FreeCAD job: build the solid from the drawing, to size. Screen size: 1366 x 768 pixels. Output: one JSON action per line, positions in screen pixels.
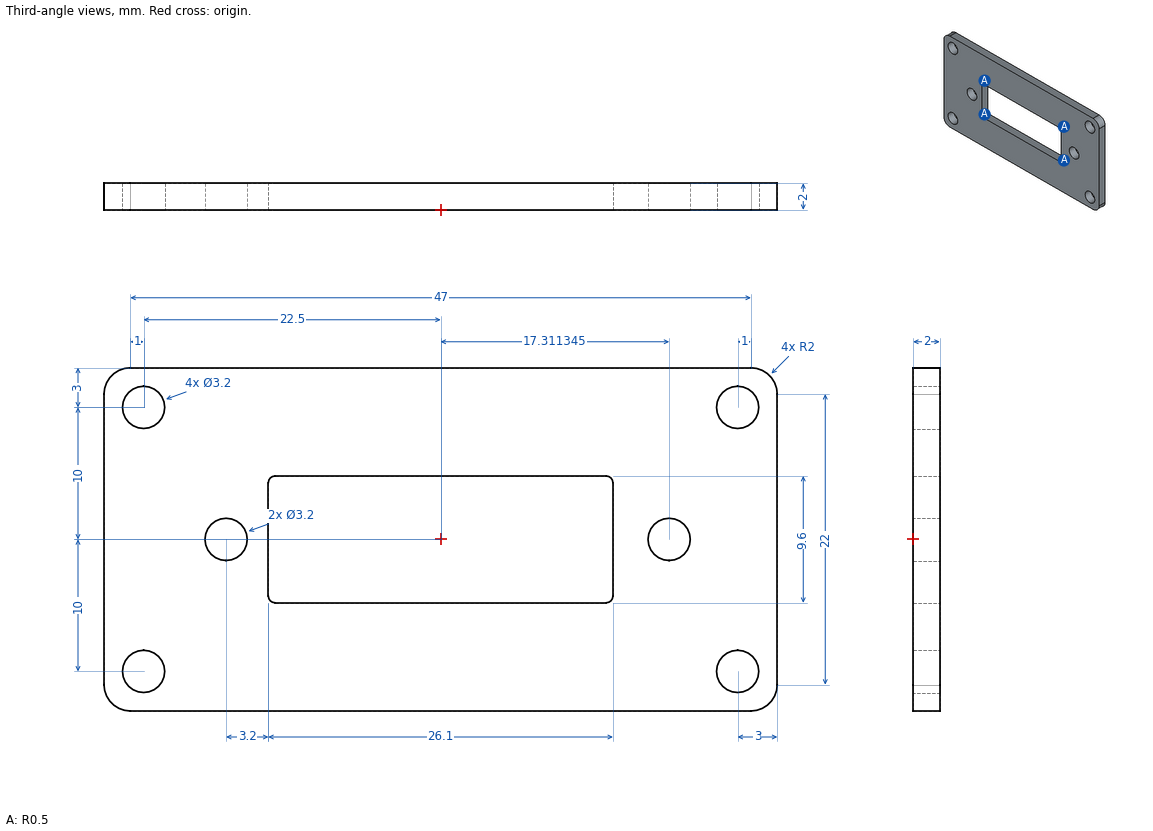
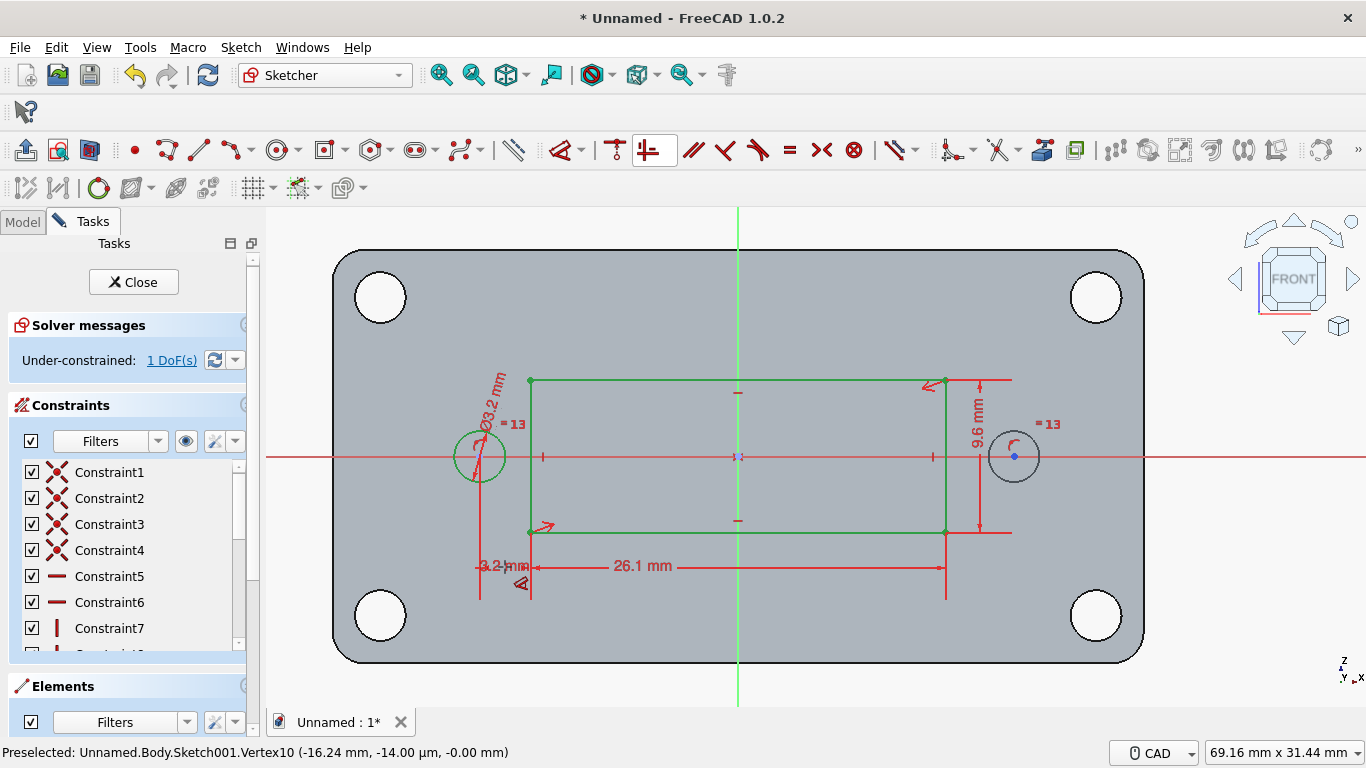
{"action": "left_click", "coordinate": [1014, 457]}
{"action": "left_click", "coordinate": [876, 491]}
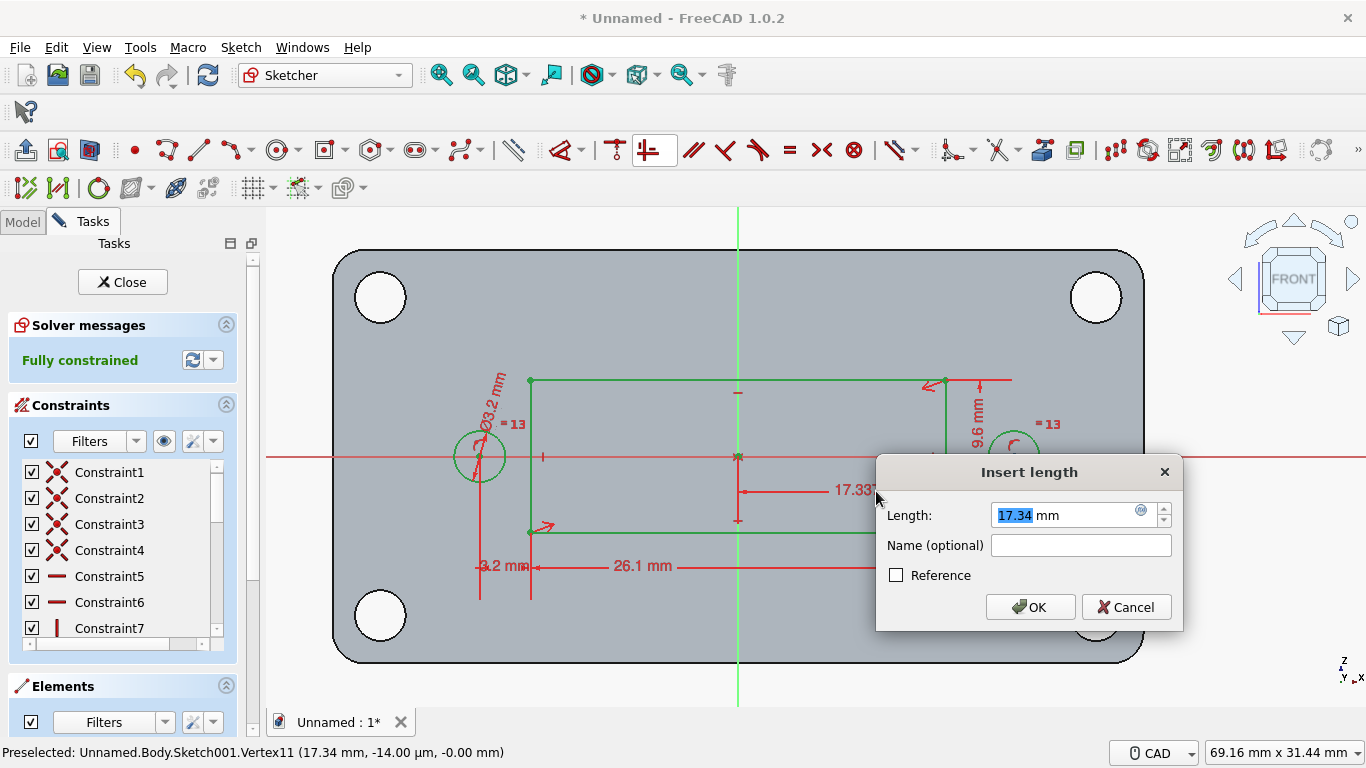
{"action": "type", "text": "17.311345"}
{"action": "key", "text": "Return"}
{"action": "key", "text": "Escape"}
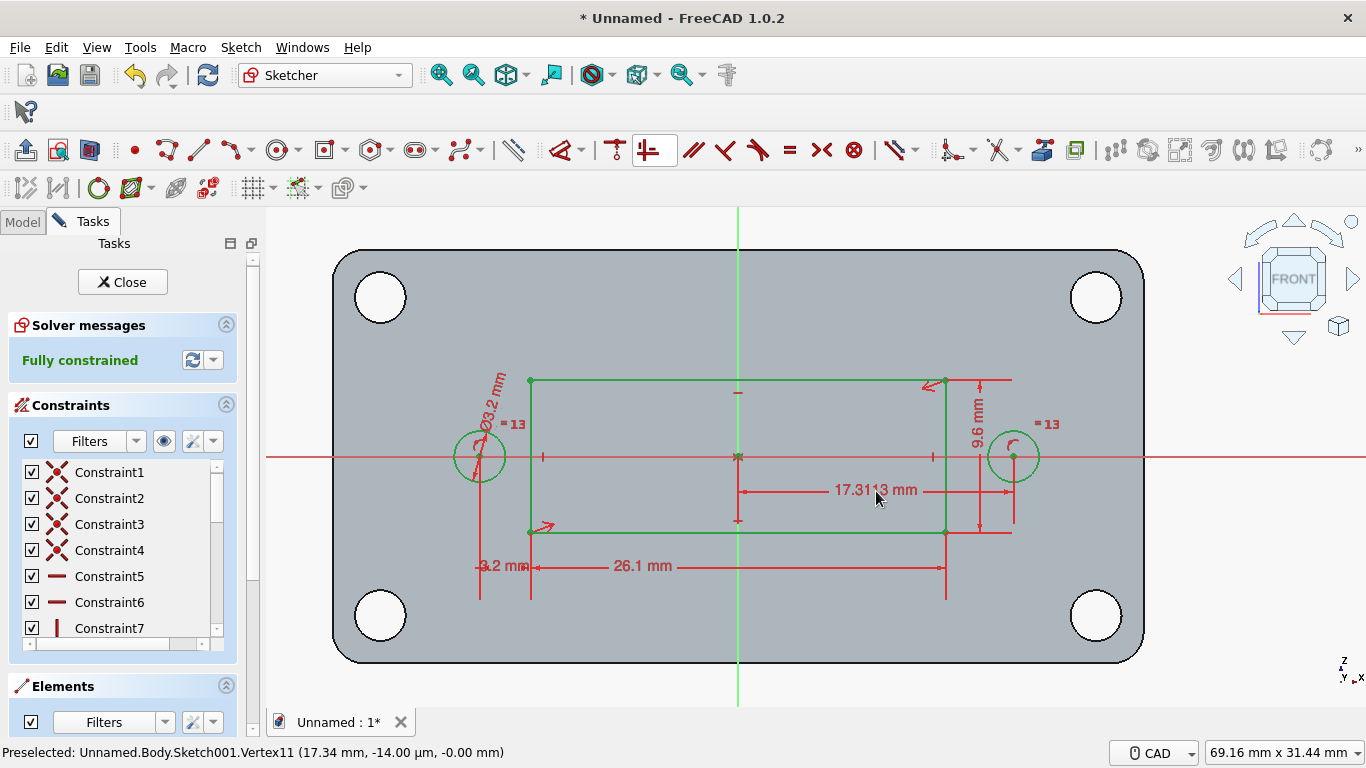
{"action": "left_click", "coordinate": [123, 282]}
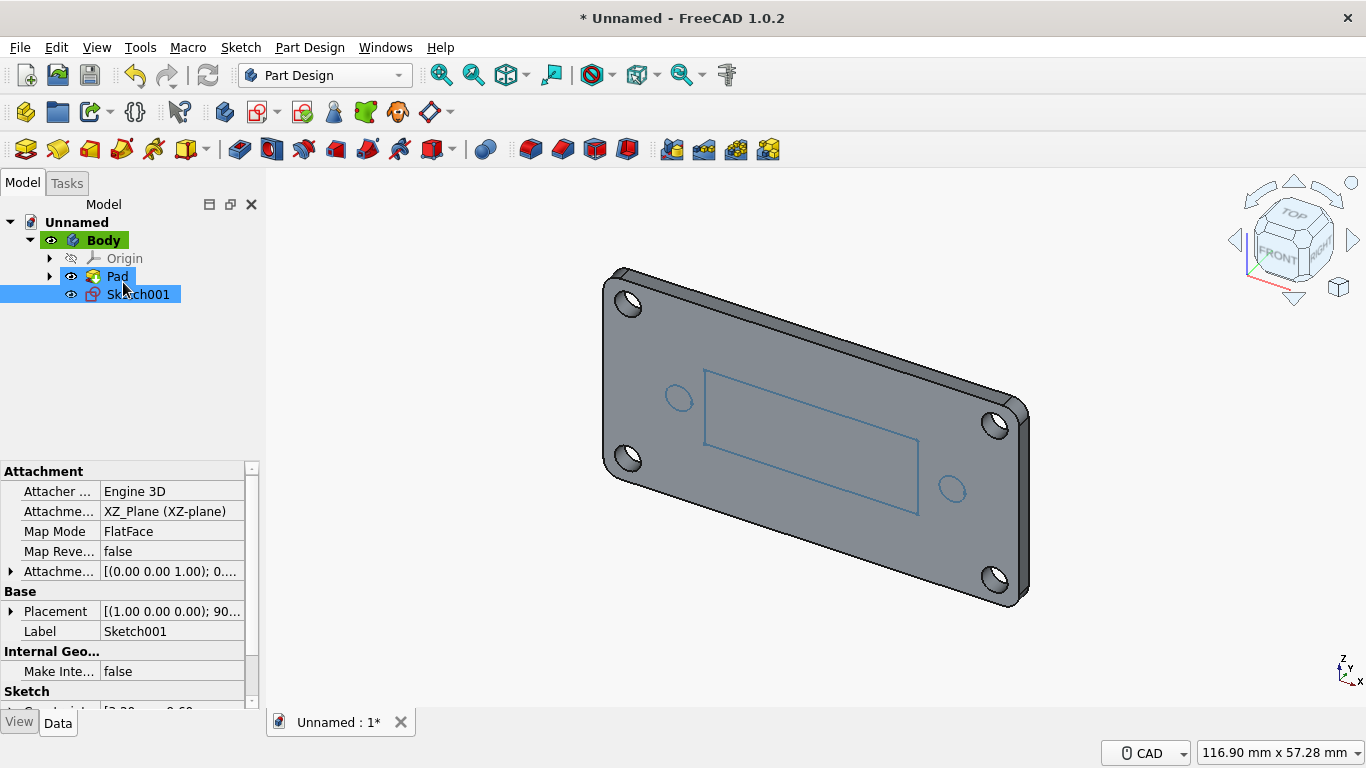
{"action": "left_click", "coordinate": [240, 150]}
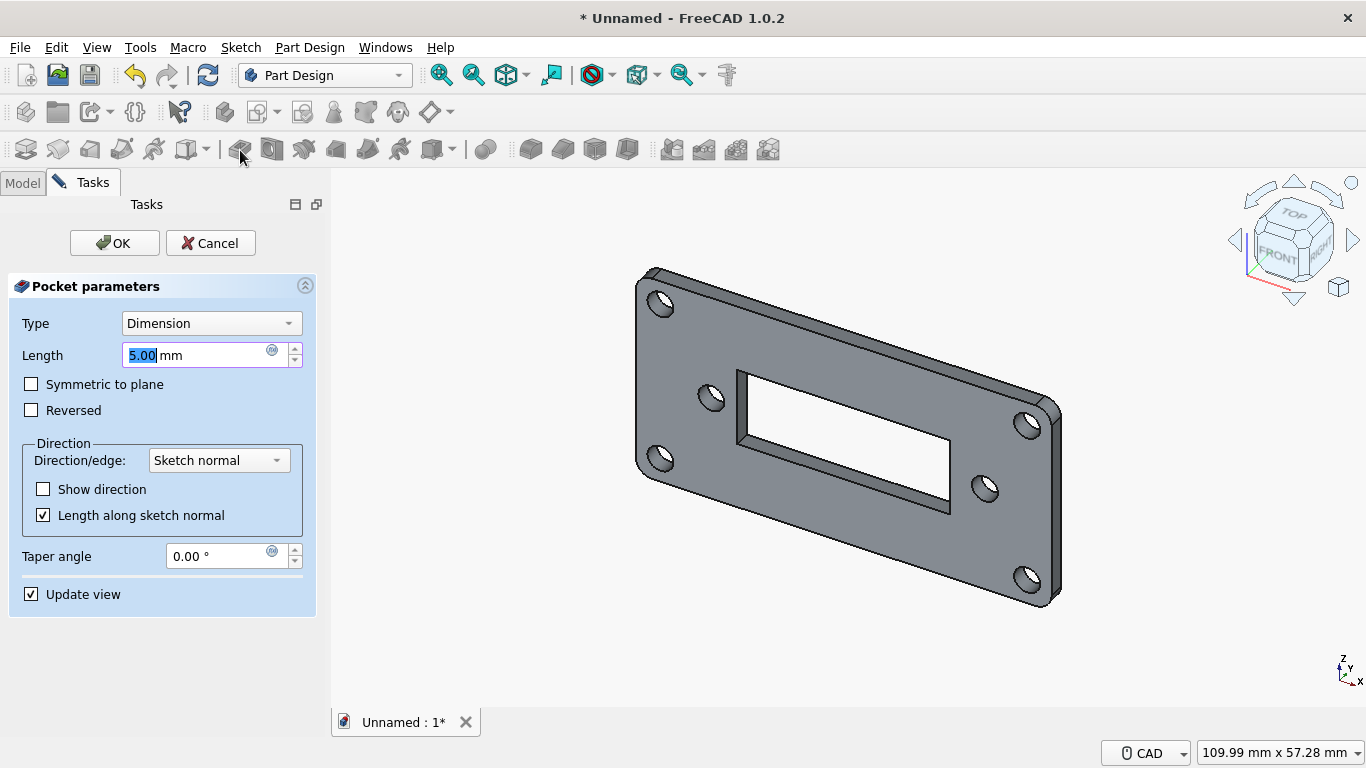
{"action": "type", "text": "2"}
{"action": "key", "text": "Tab"}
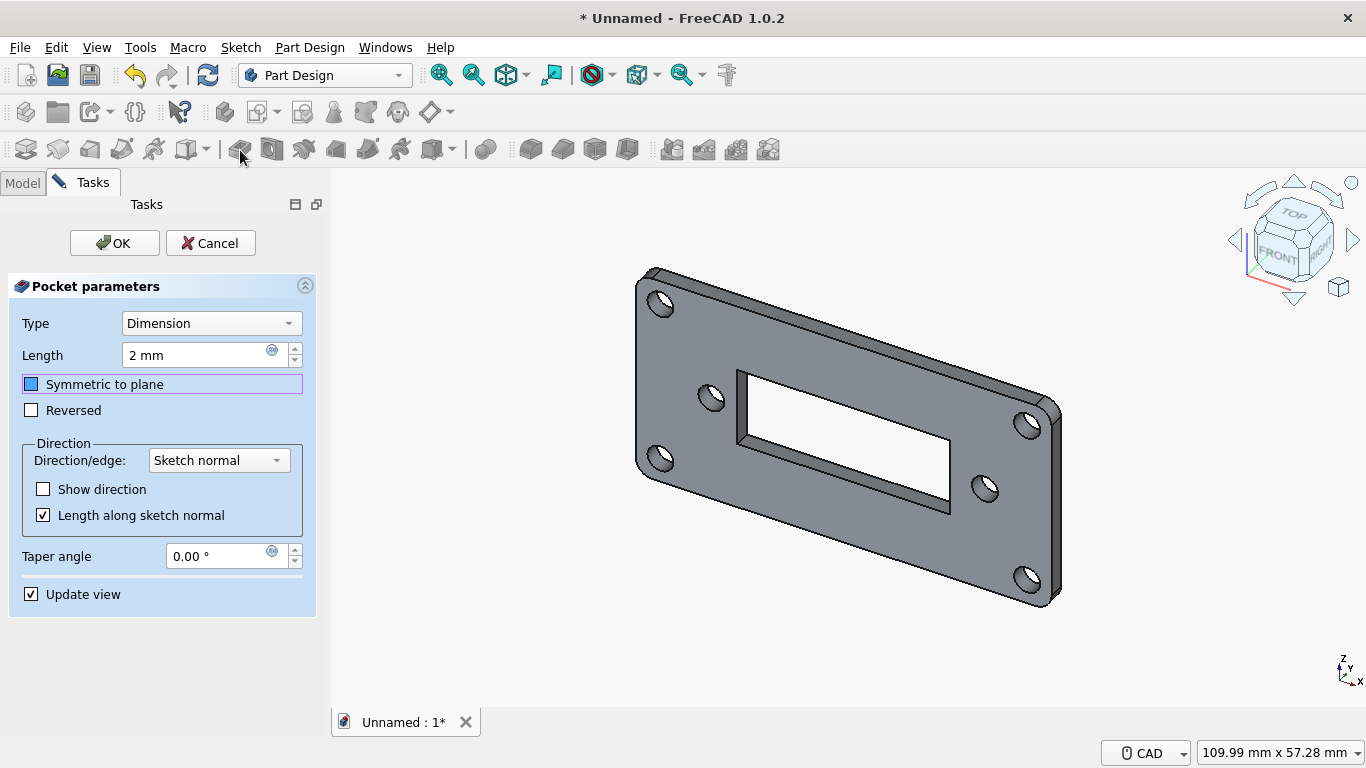
{"action": "left_click", "coordinate": [115, 243]}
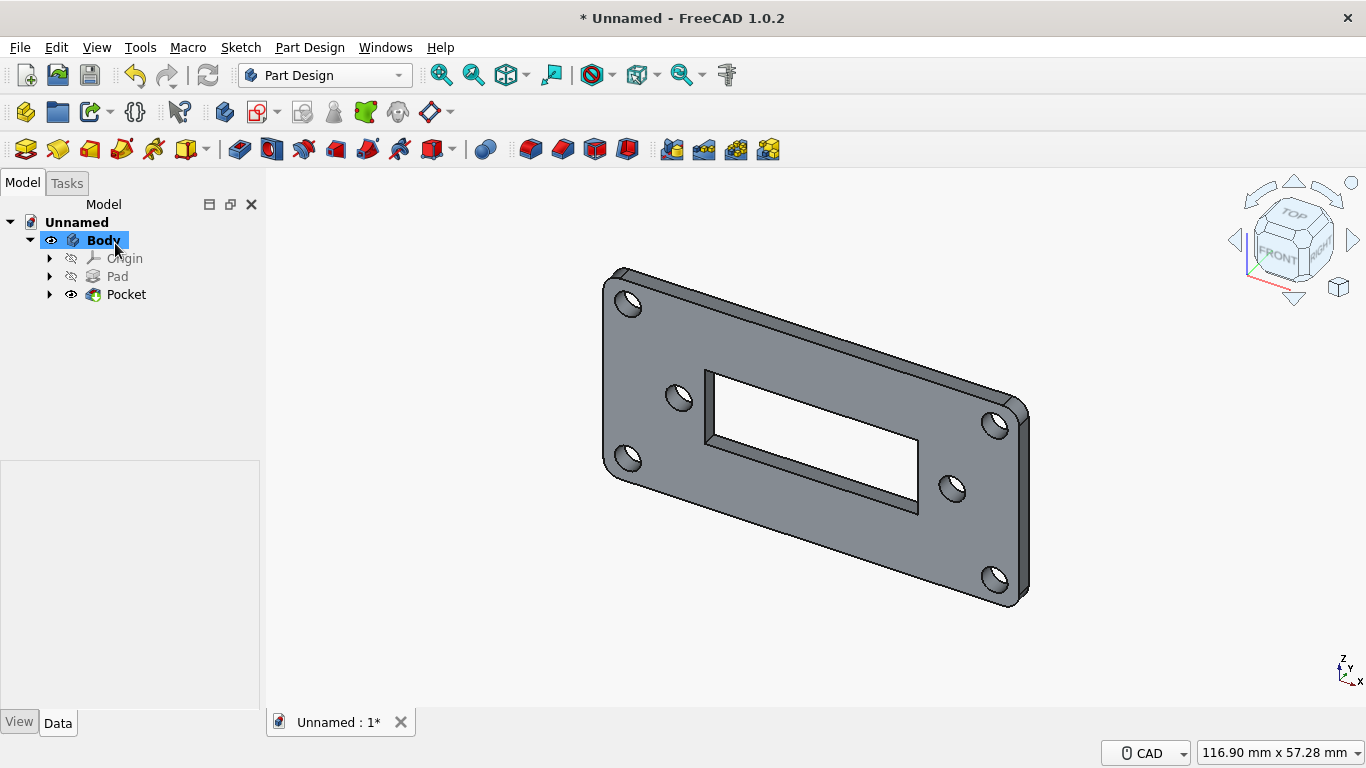
{"action": "scroll", "coordinate": [922, 435], "scroll_direction": "up", "scroll_amount": 4}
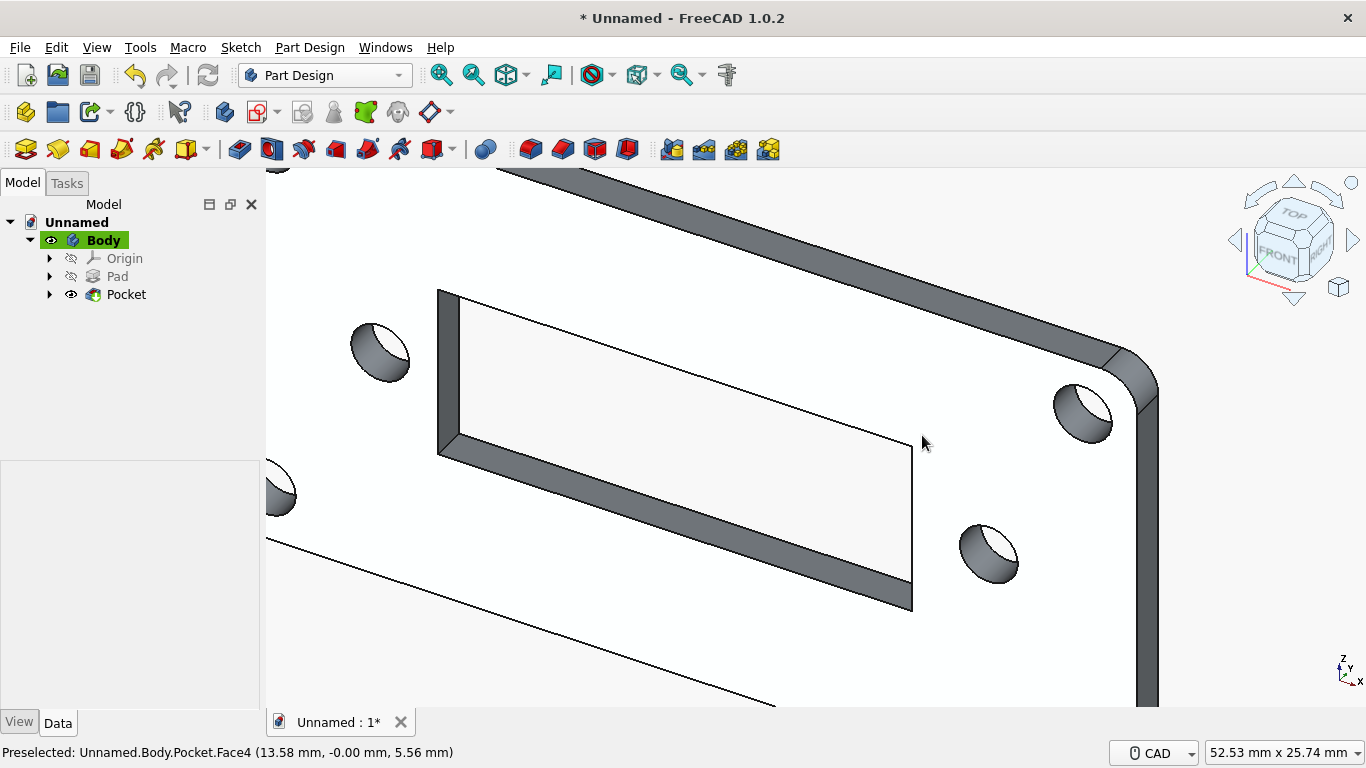
{"action": "left_click", "coordinate": [442, 76]}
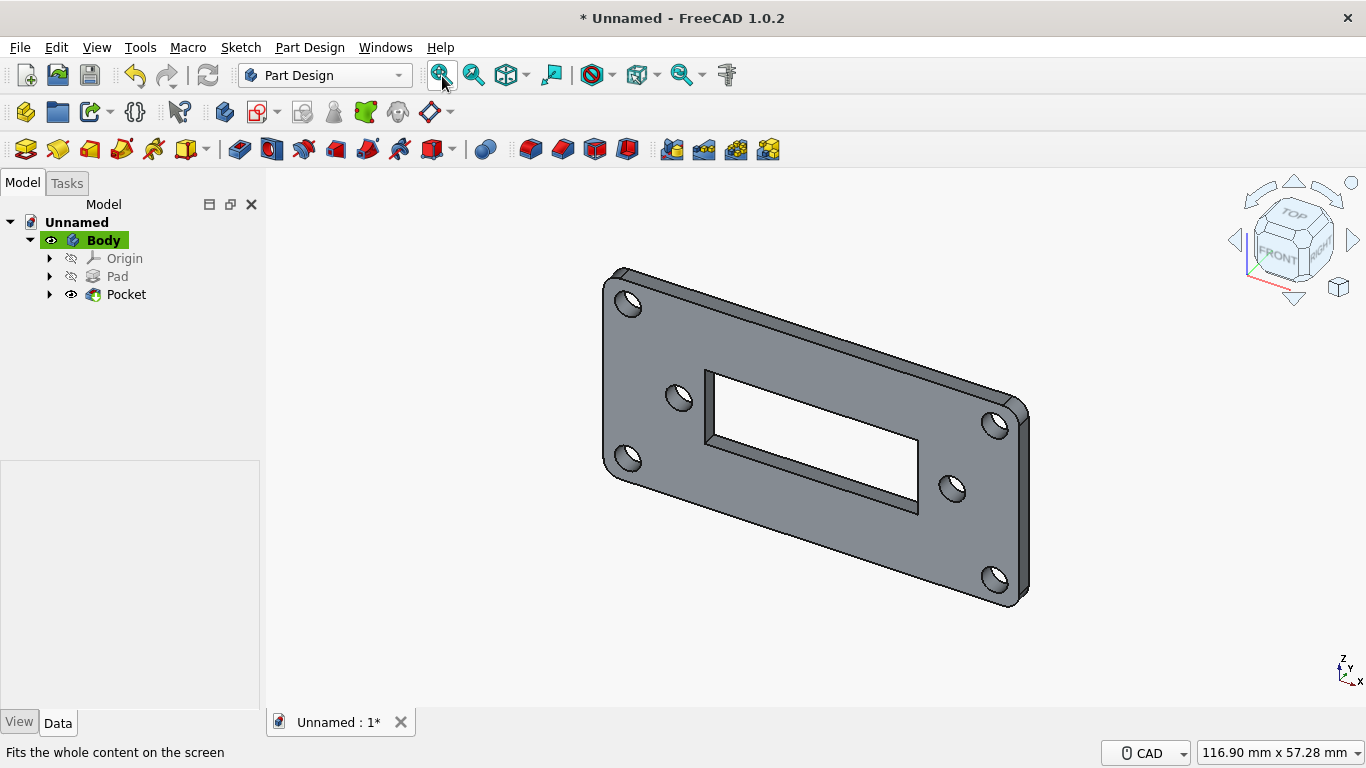
{"action": "key", "text": "0"}